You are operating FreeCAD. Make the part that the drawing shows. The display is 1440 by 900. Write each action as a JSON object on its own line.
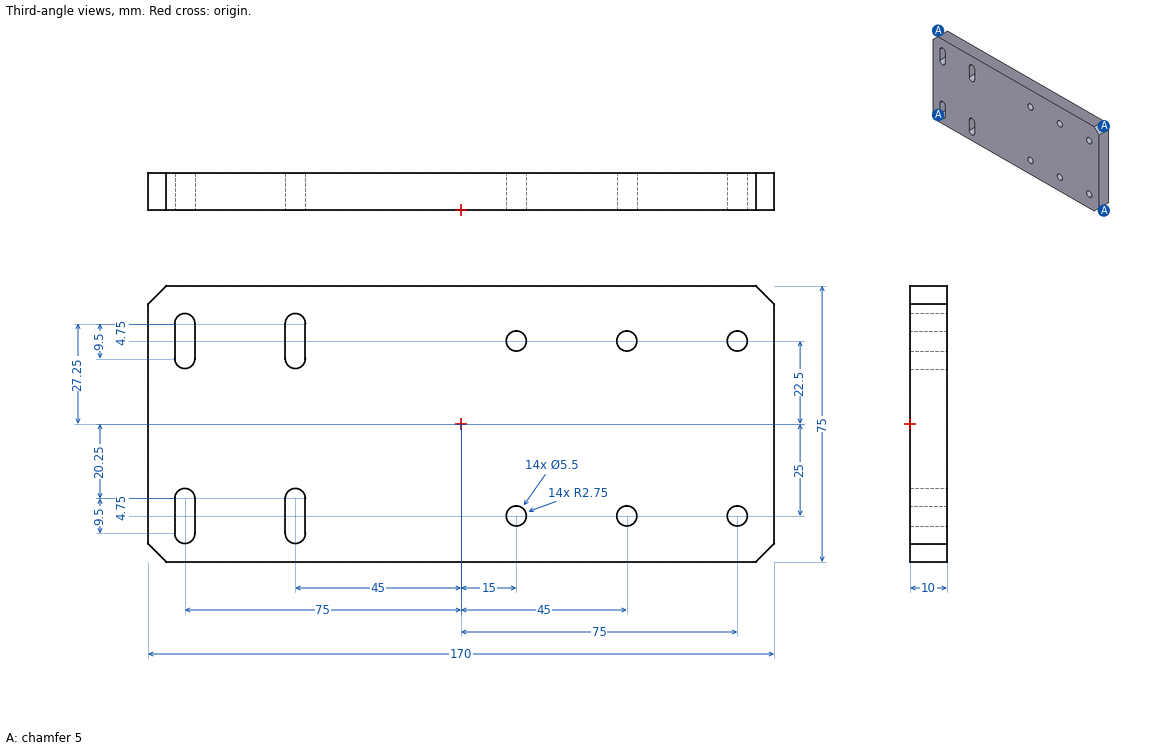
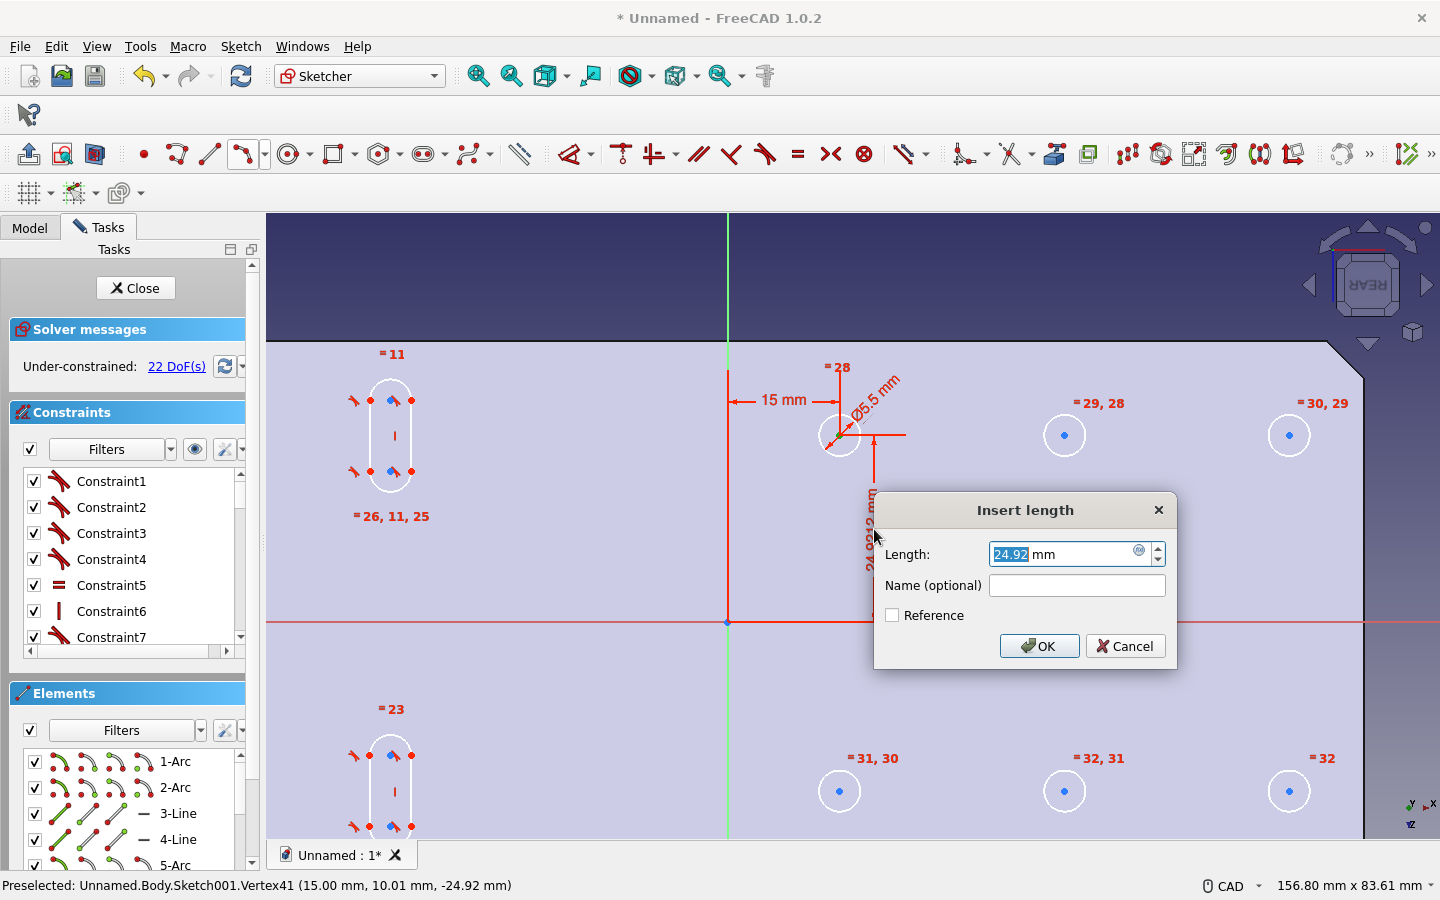
{"action": "type", "text": "25"}
{"action": "key", "text": "Return"}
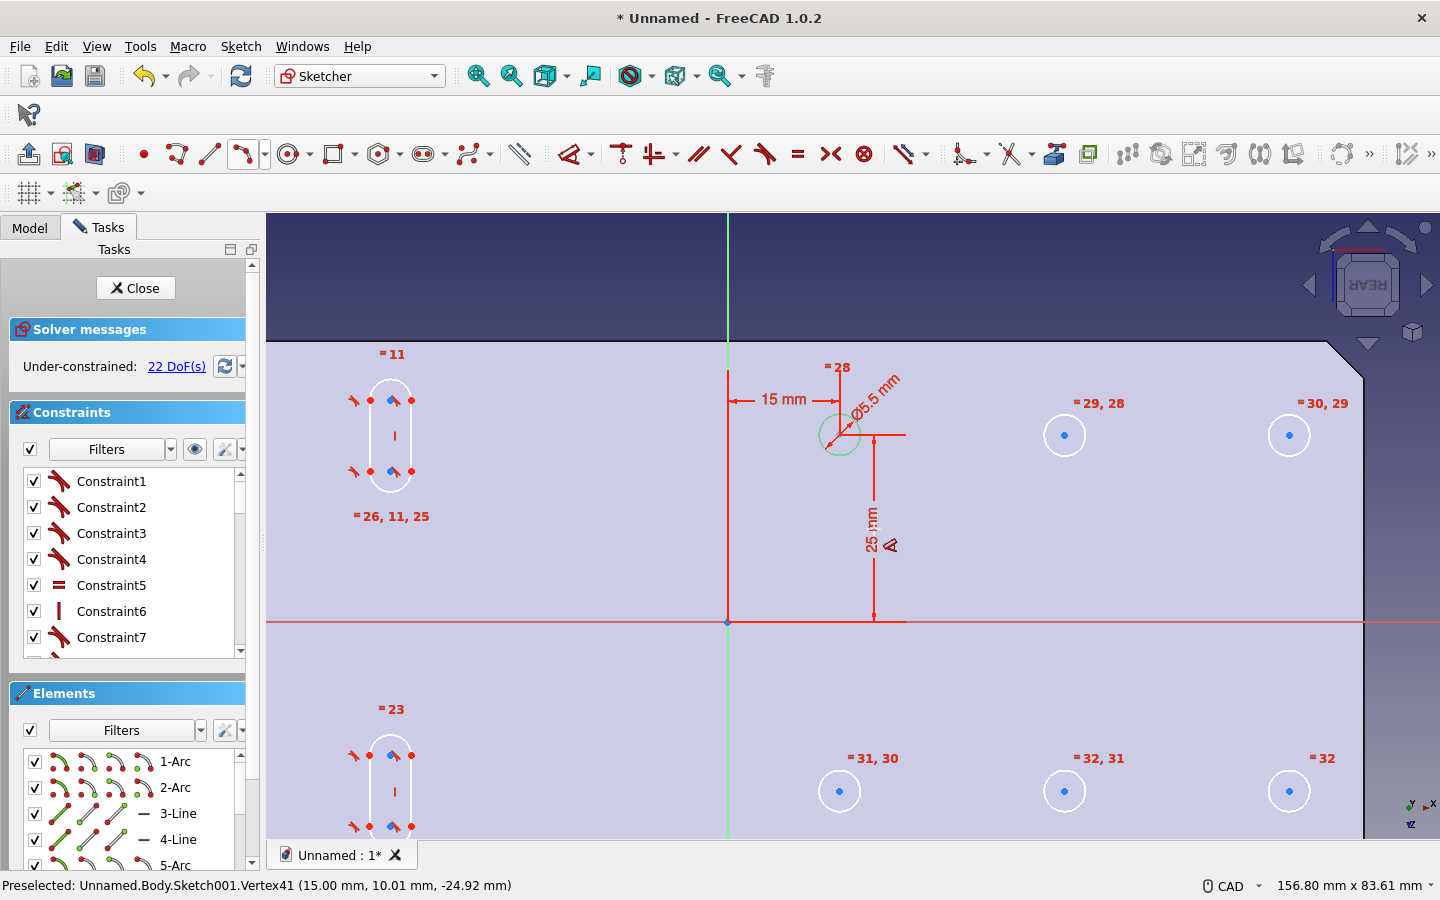
{"action": "left_click", "coordinate": [1065, 435]}
{"action": "left_click", "coordinate": [974, 401]}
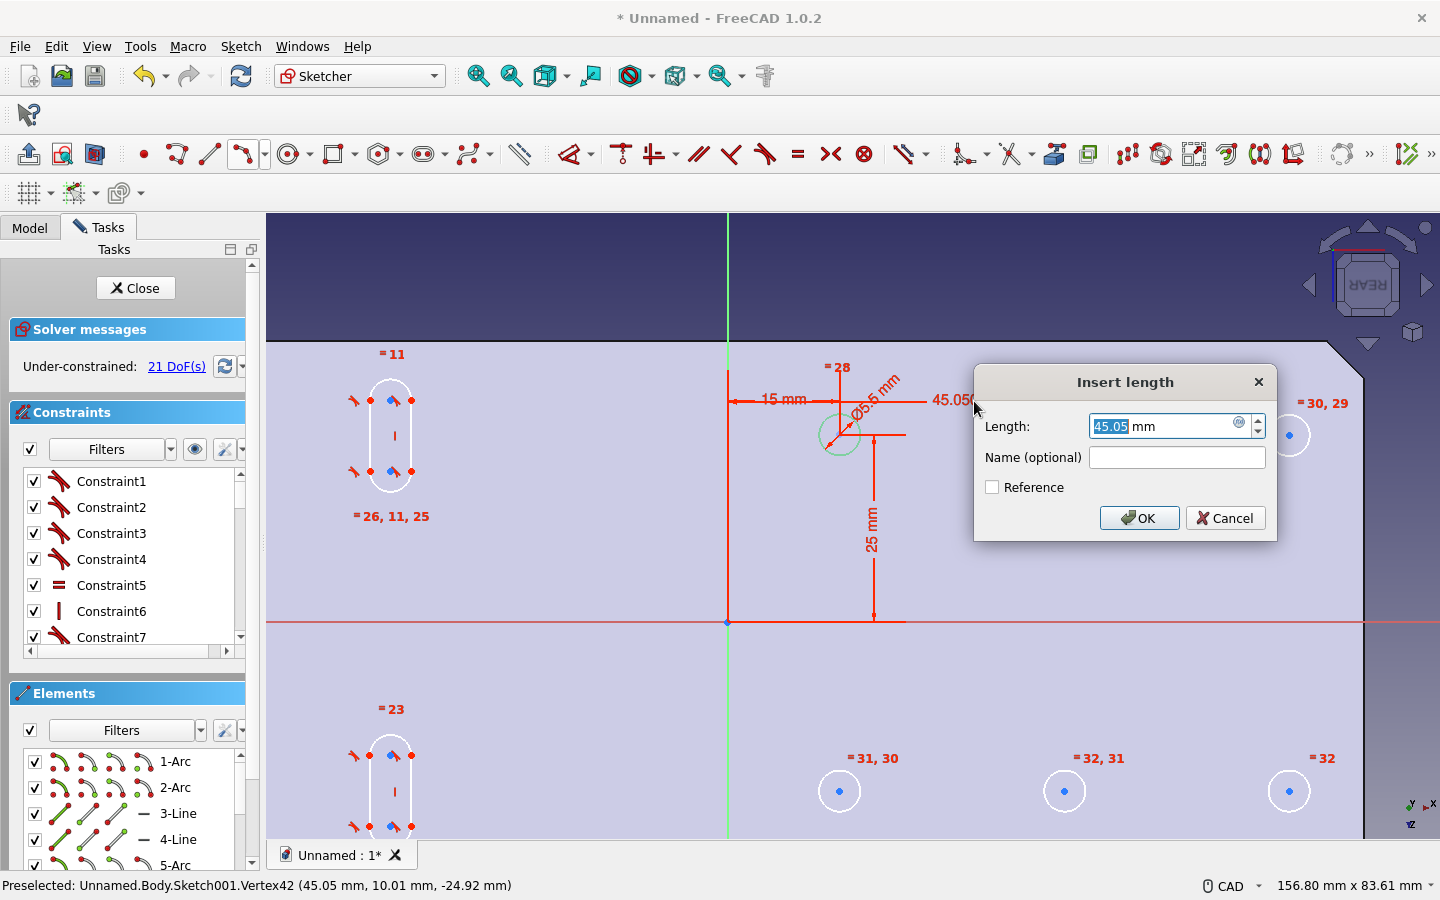
{"action": "type", "text": "45"}
{"action": "key", "text": "Return"}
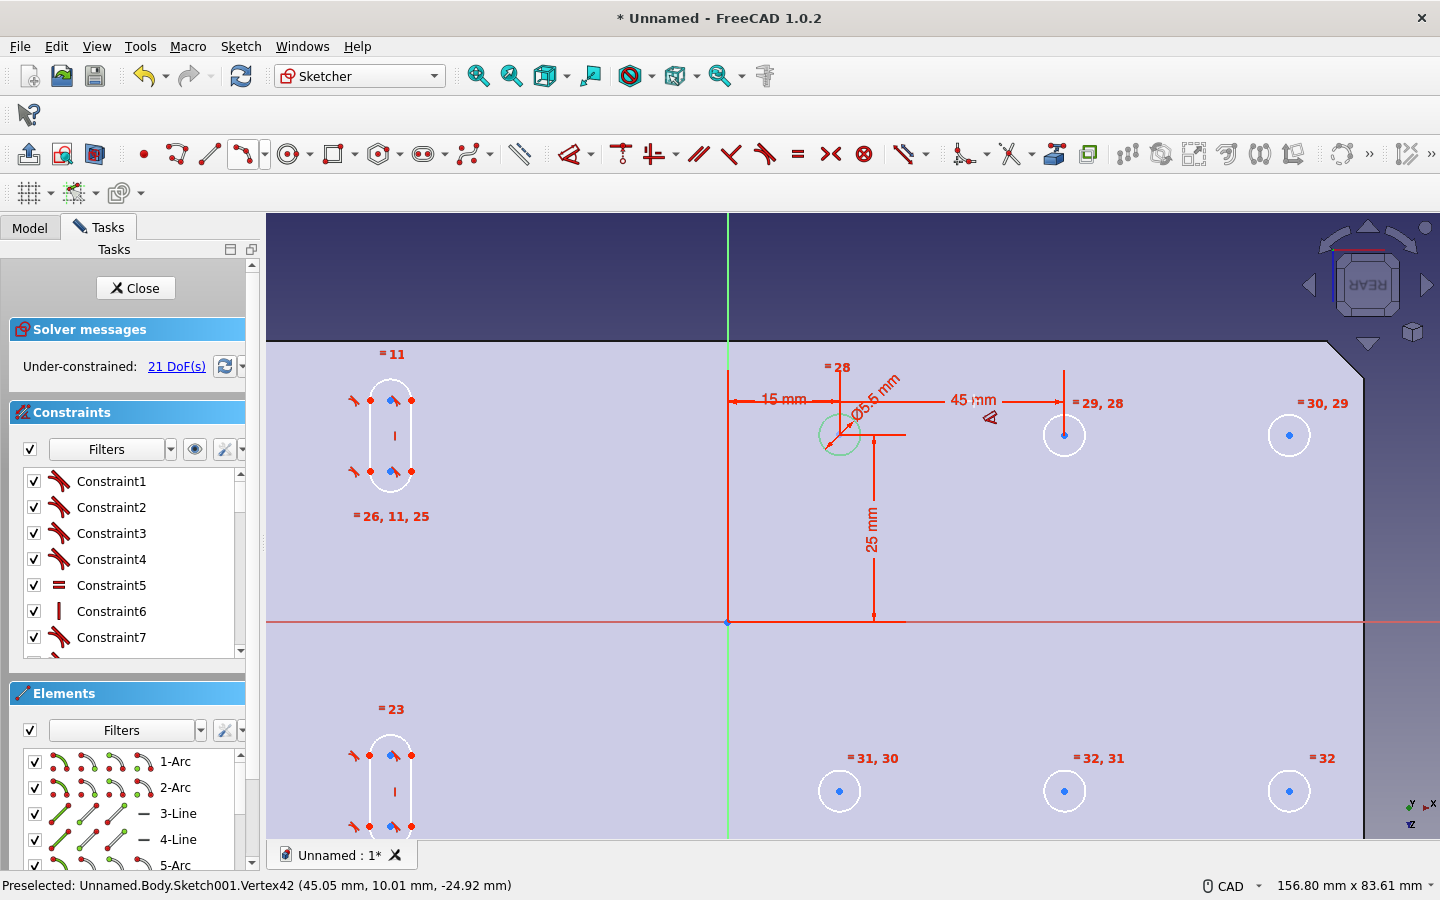
{"action": "left_click", "coordinate": [1064, 435]}
{"action": "left_click", "coordinate": [1098, 529]}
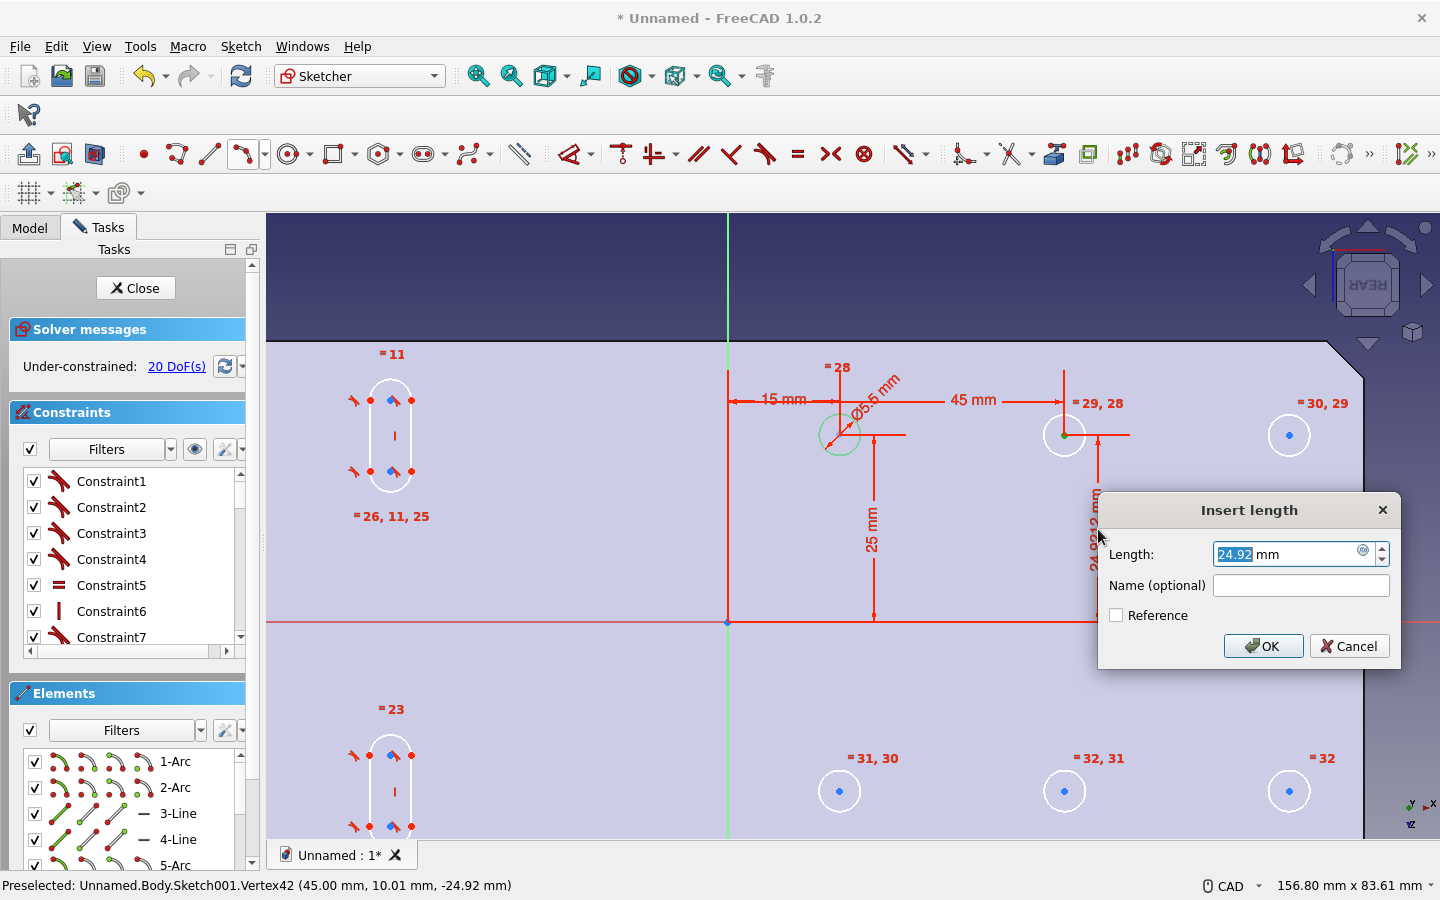
{"action": "type", "text": "25"}
{"action": "key", "text": "Return"}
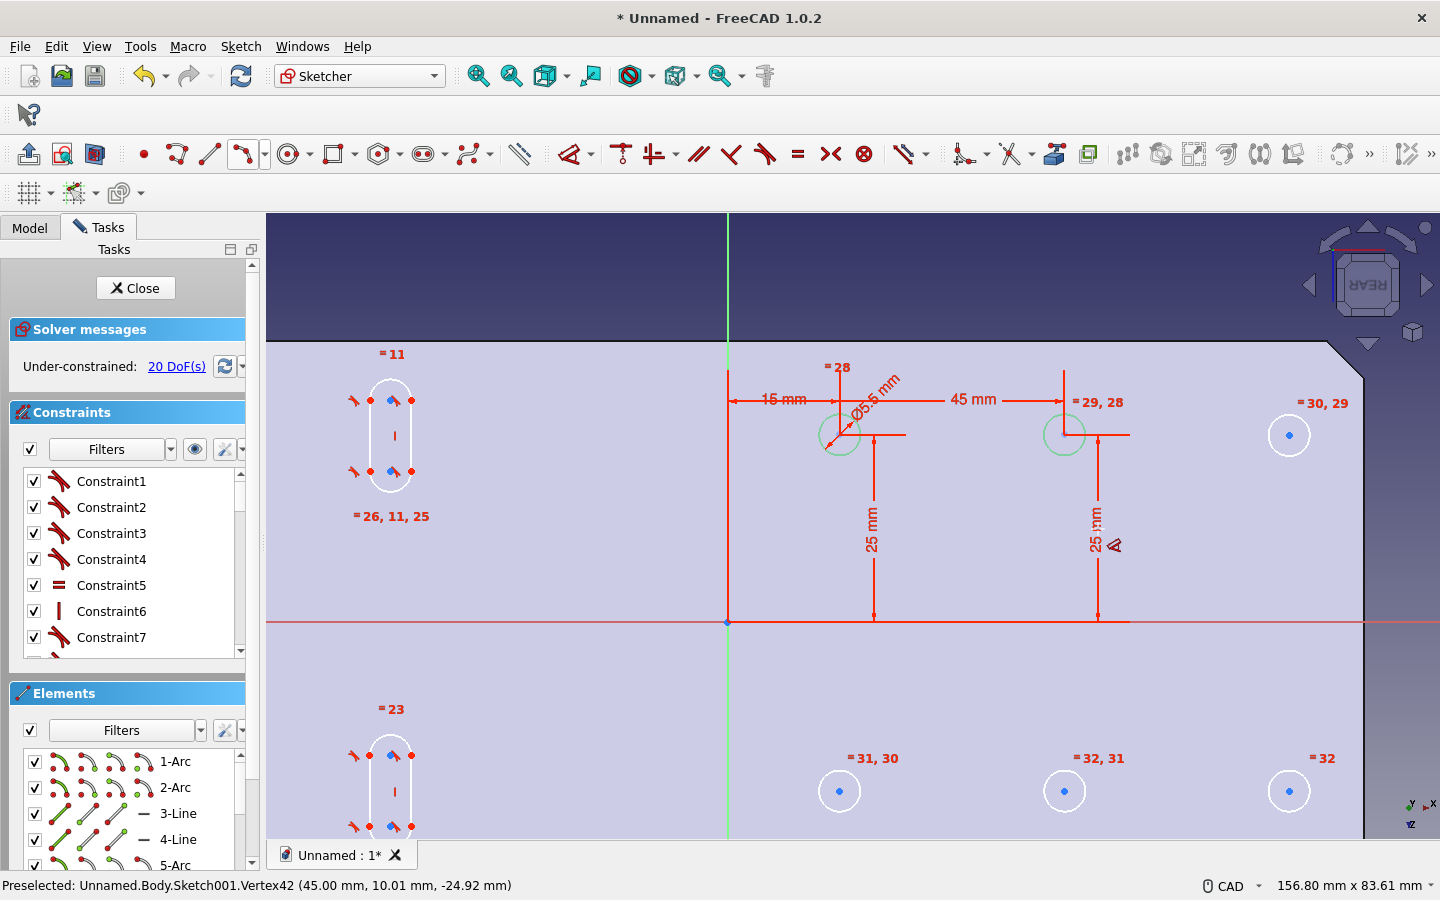
{"action": "scroll", "coordinate": [854, 421], "scroll_direction": "down", "scroll_amount": 3}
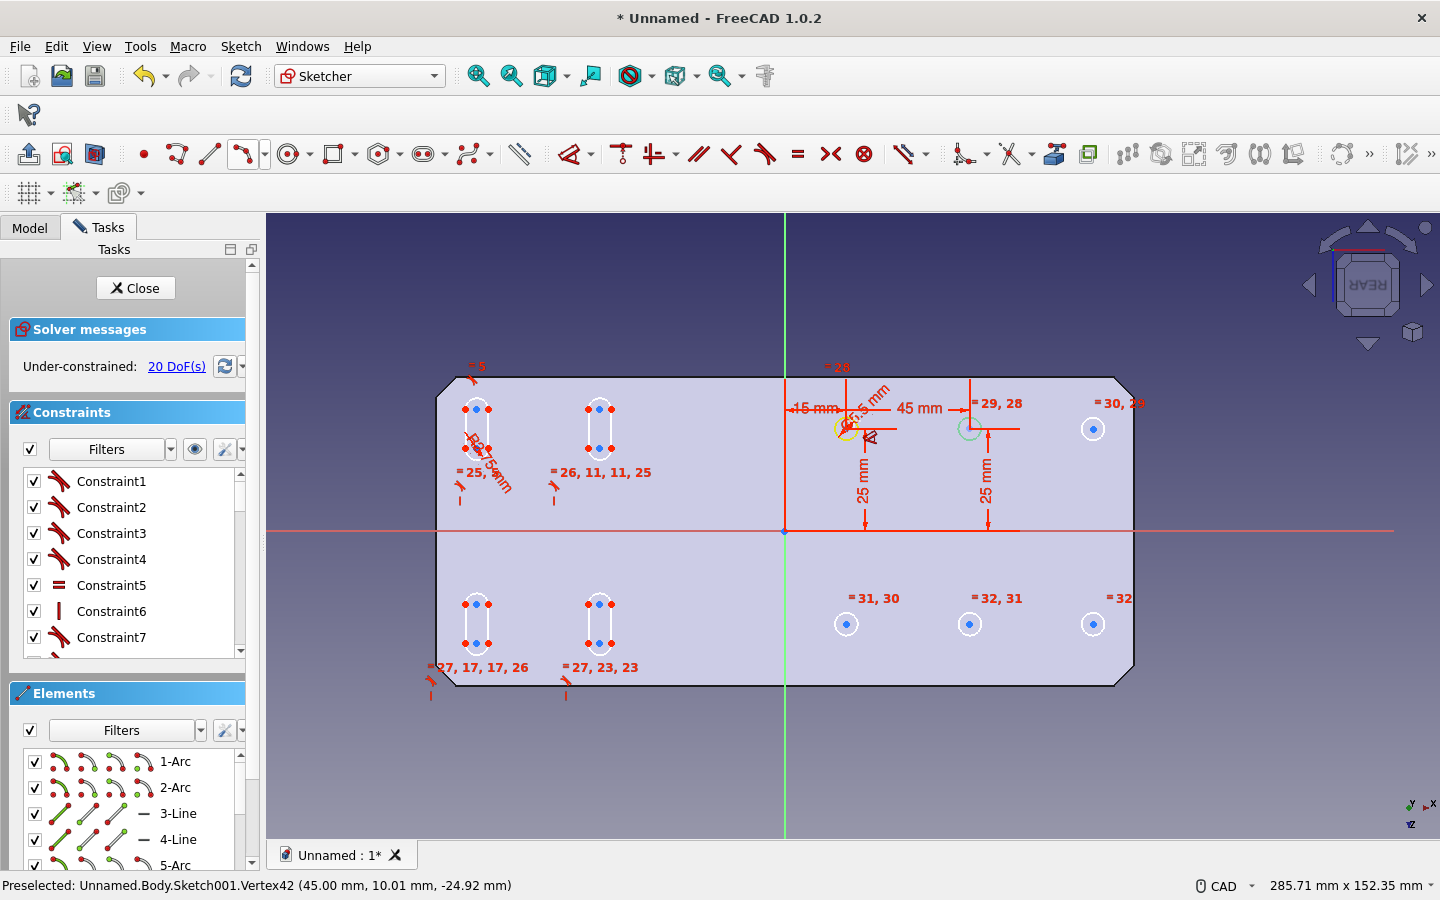
{"action": "left_click", "coordinate": [1093, 429]}
{"action": "left_click", "coordinate": [1010, 395]}